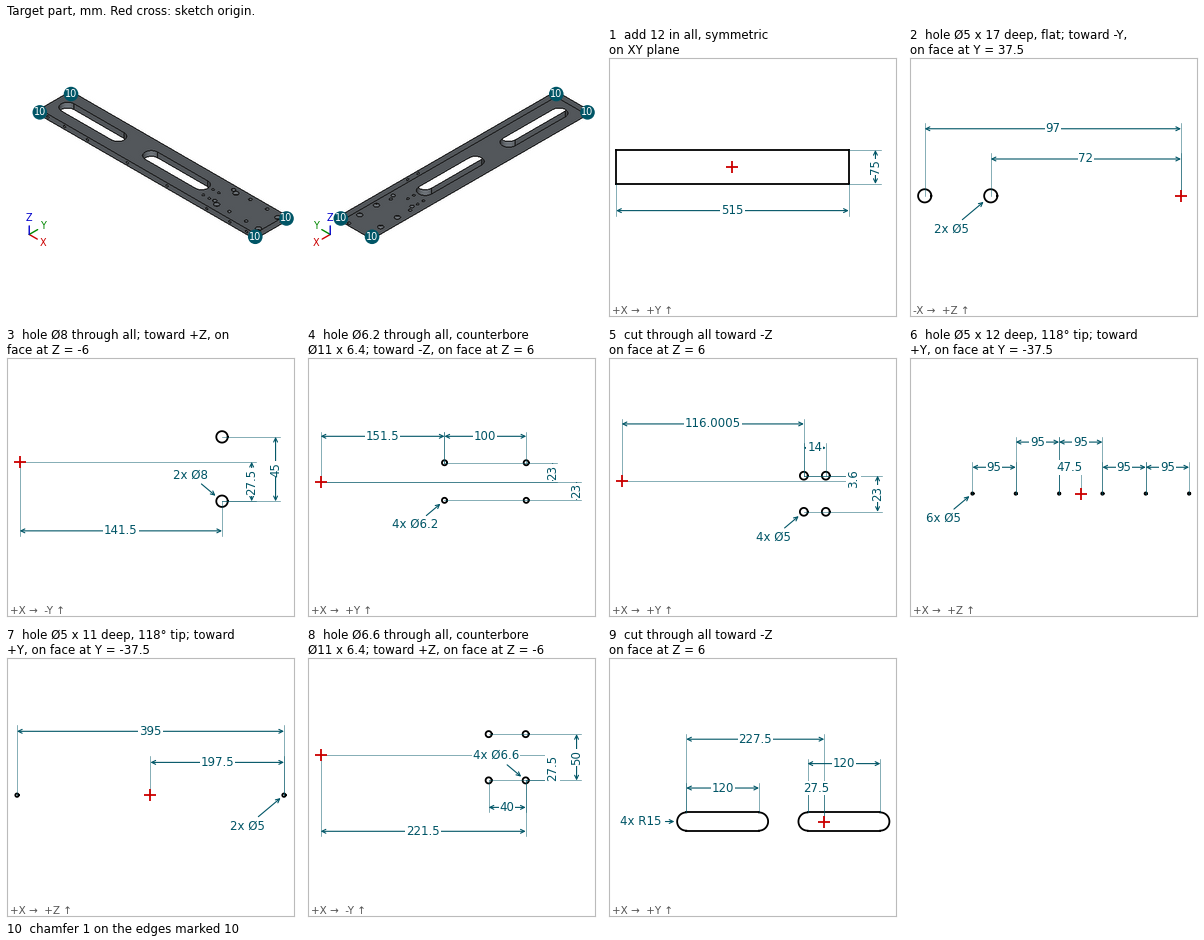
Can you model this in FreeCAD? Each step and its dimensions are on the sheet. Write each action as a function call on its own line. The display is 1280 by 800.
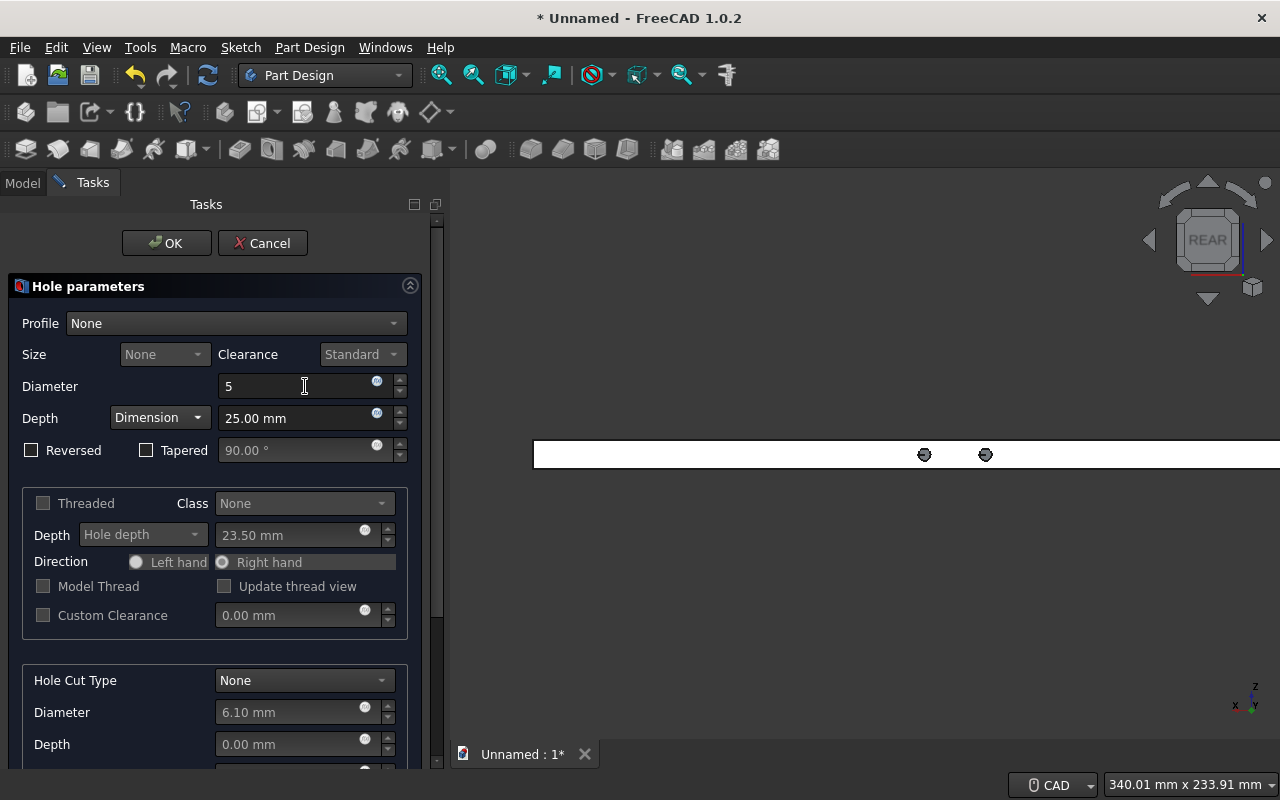
triple_click(305, 418)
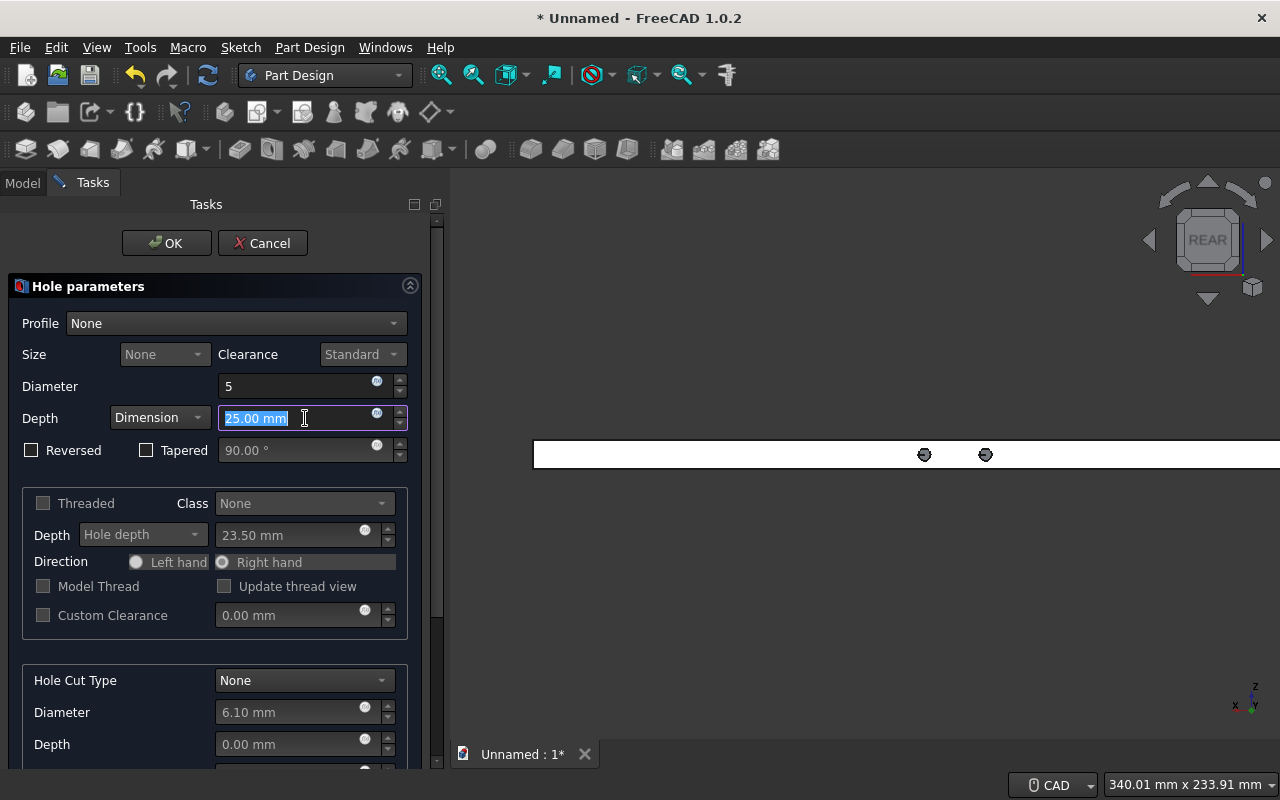
text(17)
key(Tab)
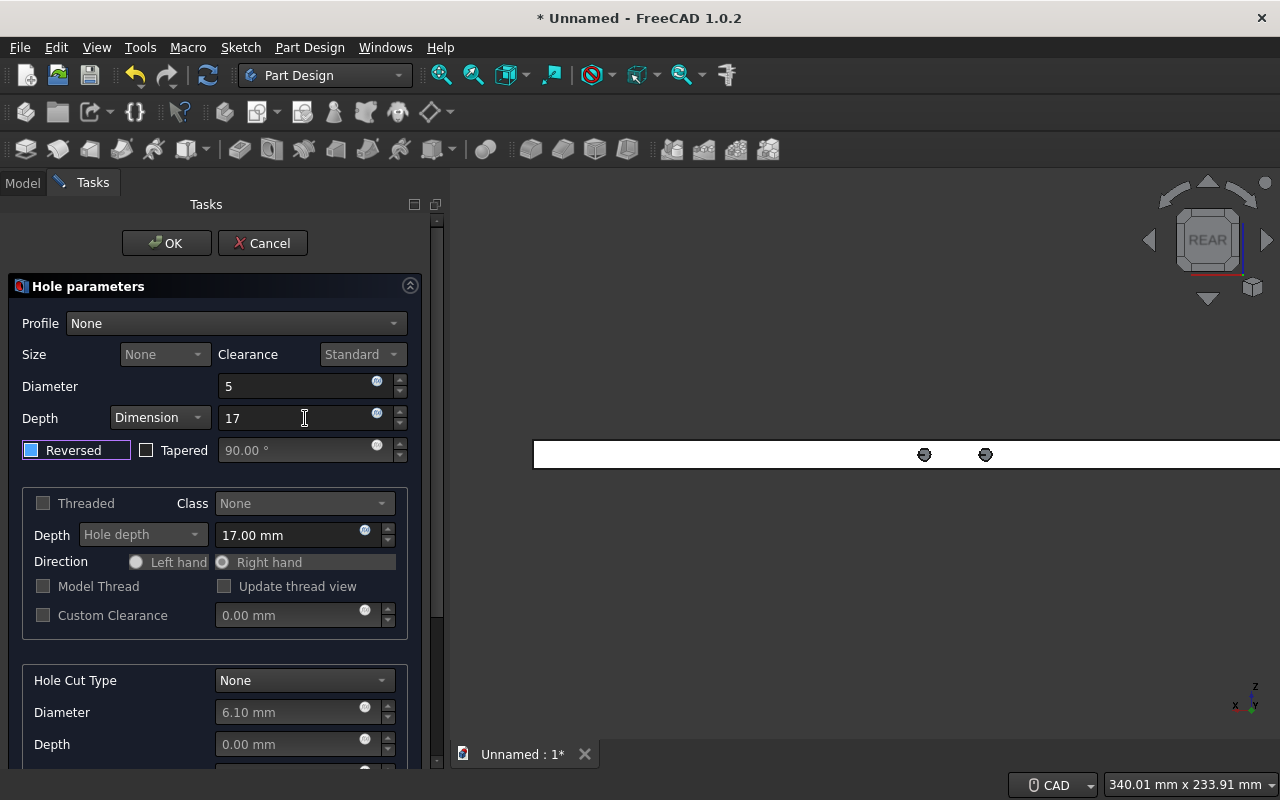
scroll(437, 491, down, 3)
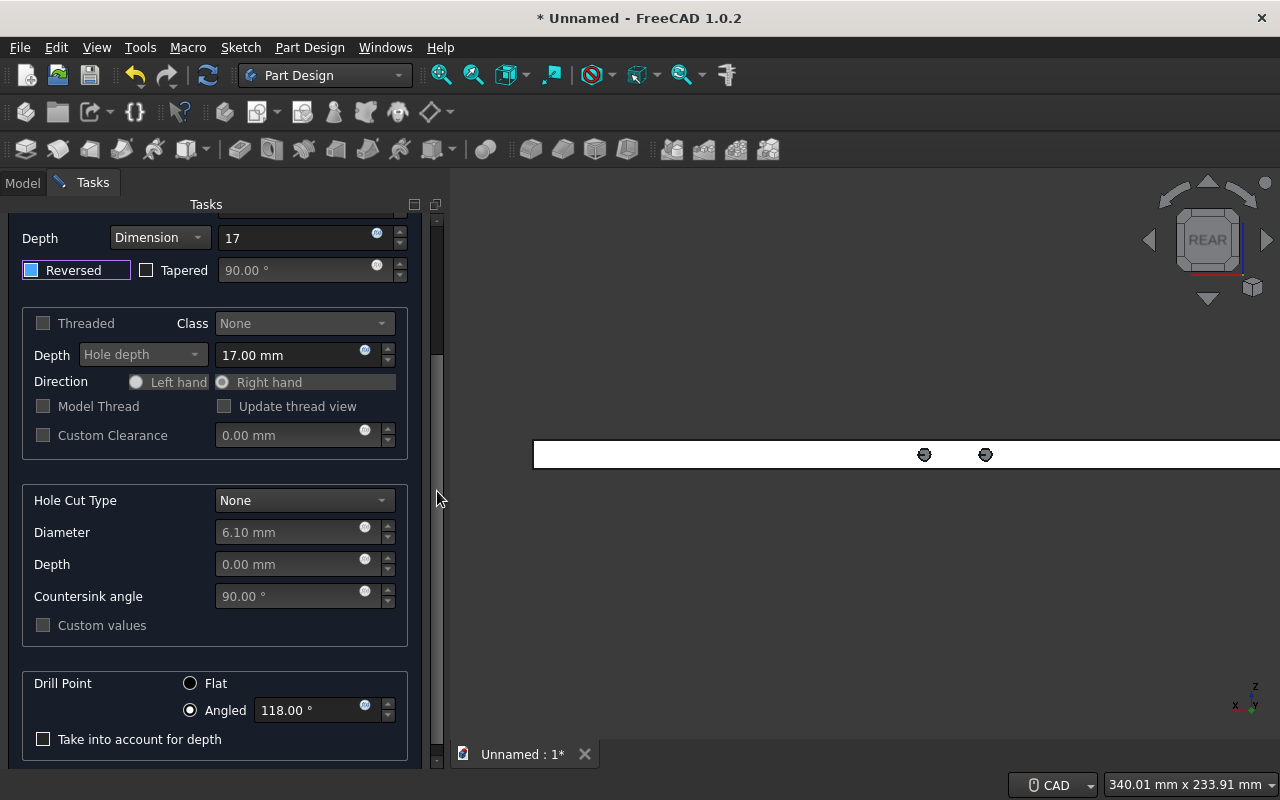
click(191, 683)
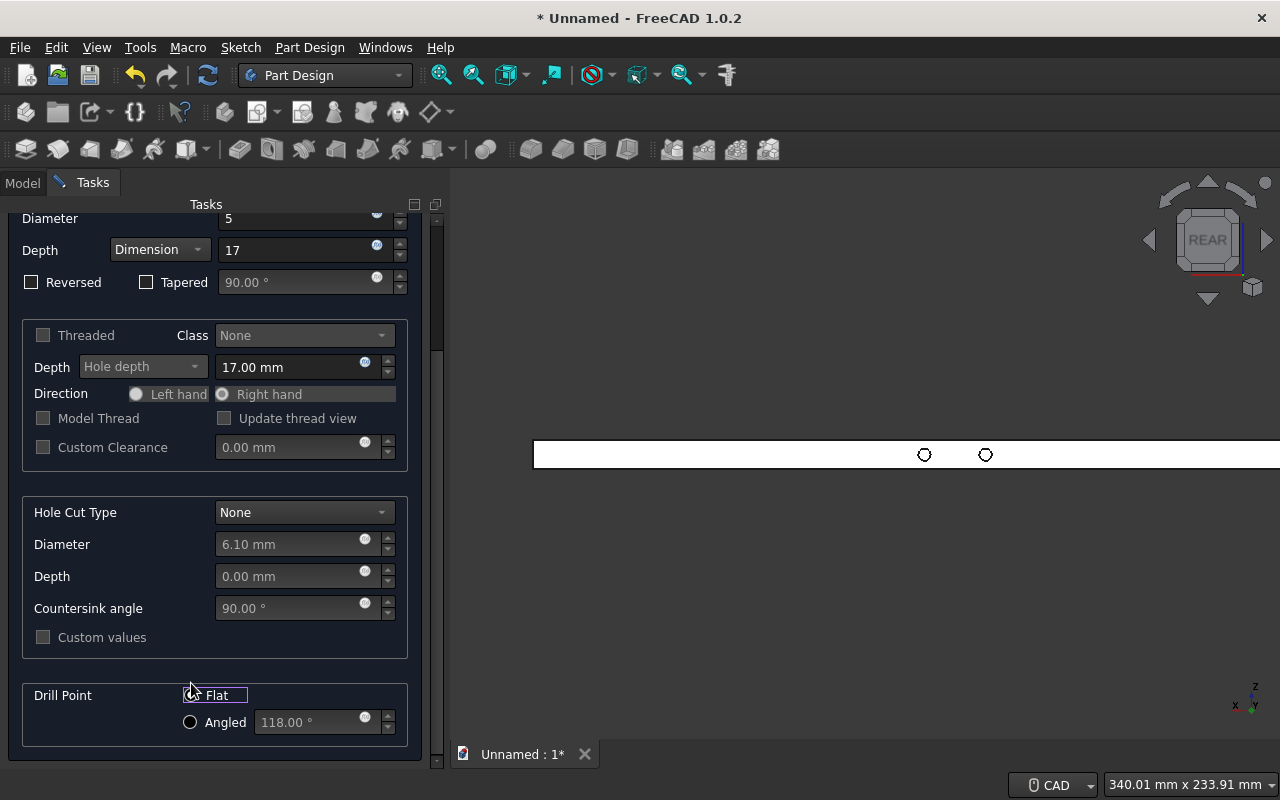
scroll(437, 491, up, 4)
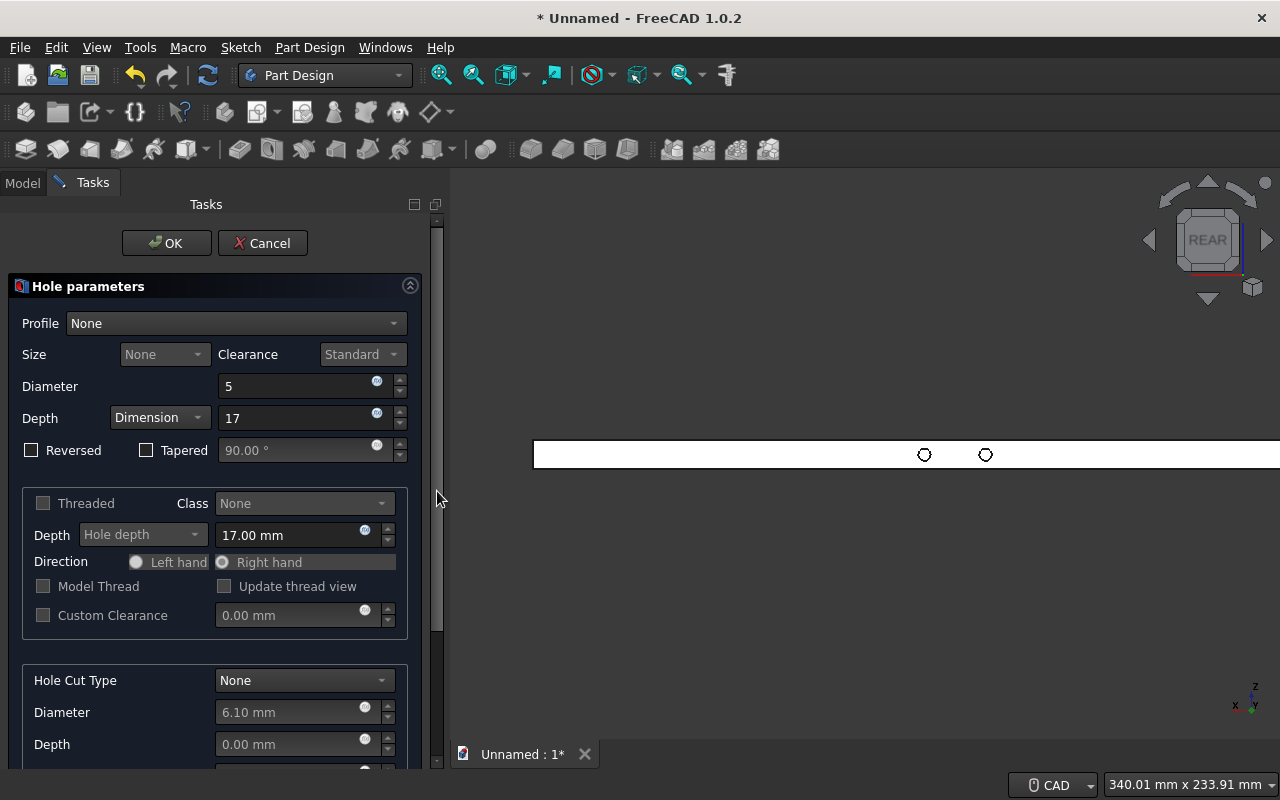
click(167, 243)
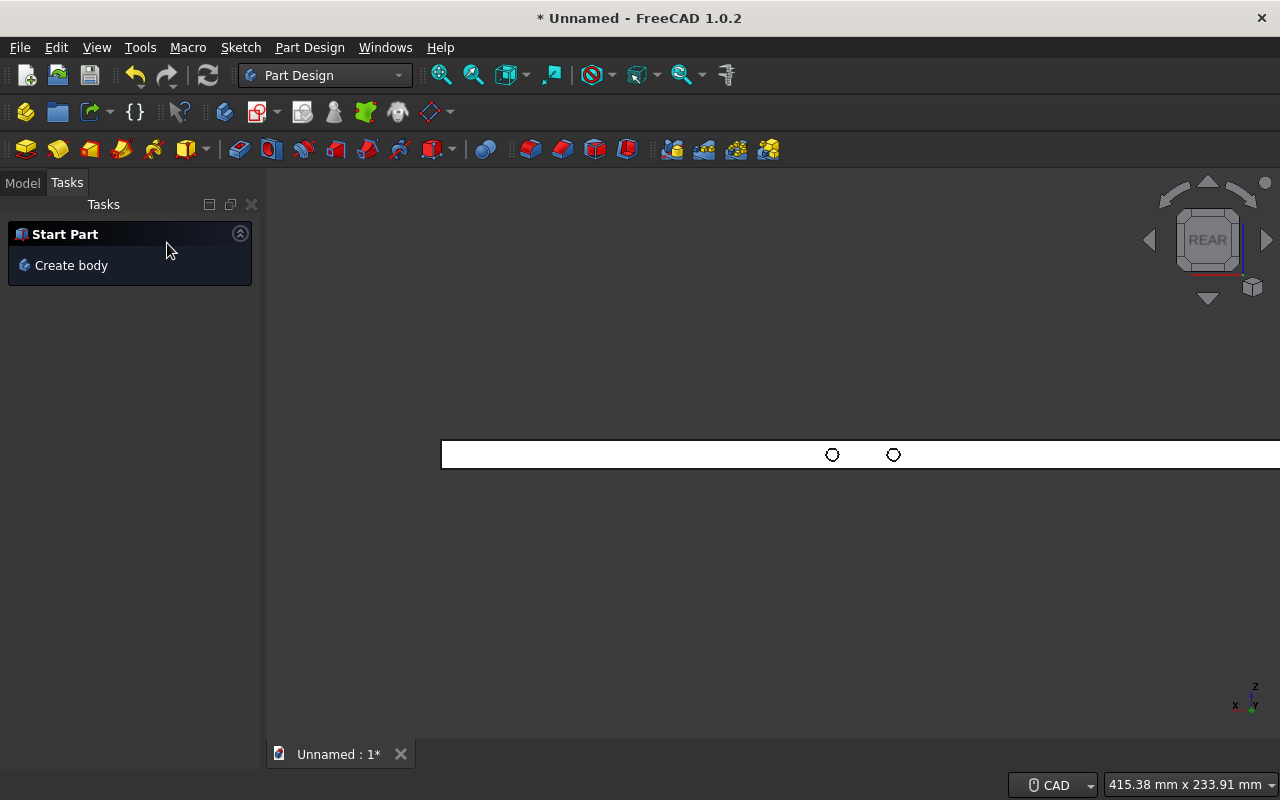
key(v)
key(f)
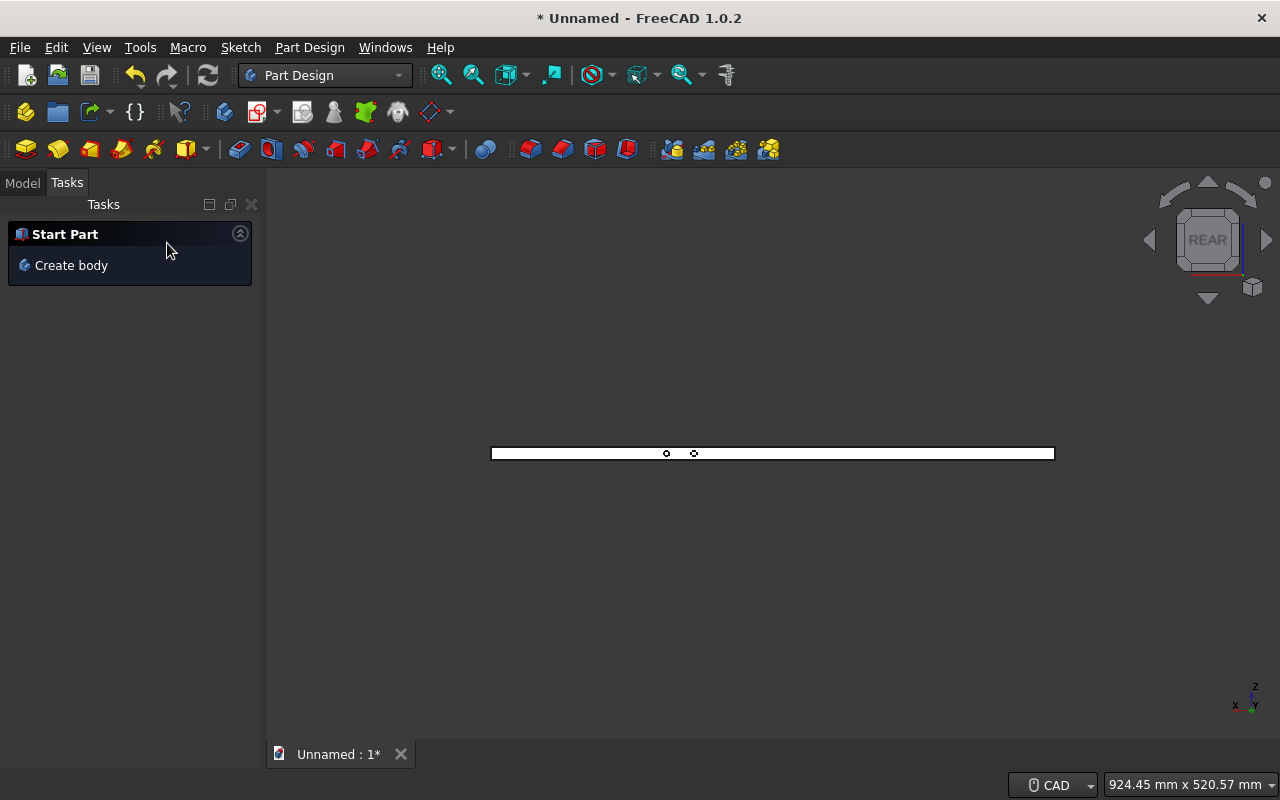
key(5)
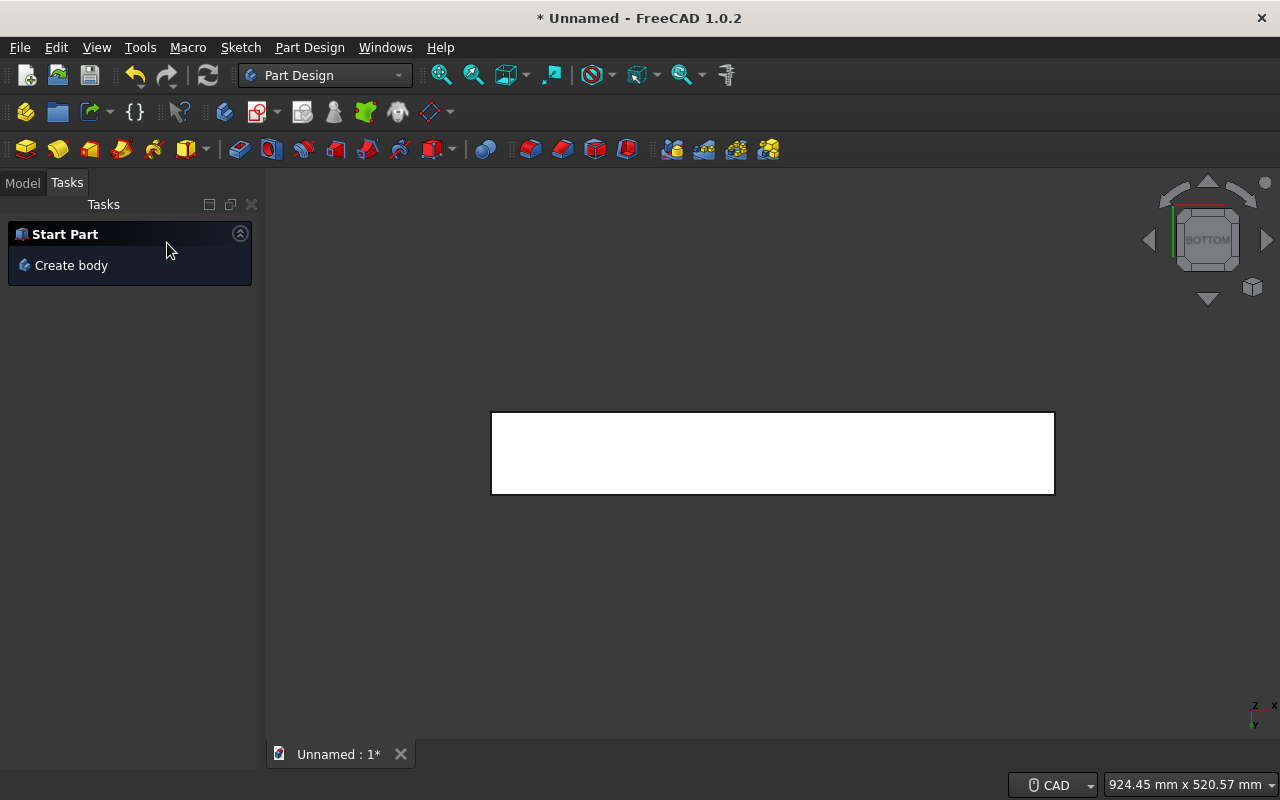
click(934, 452)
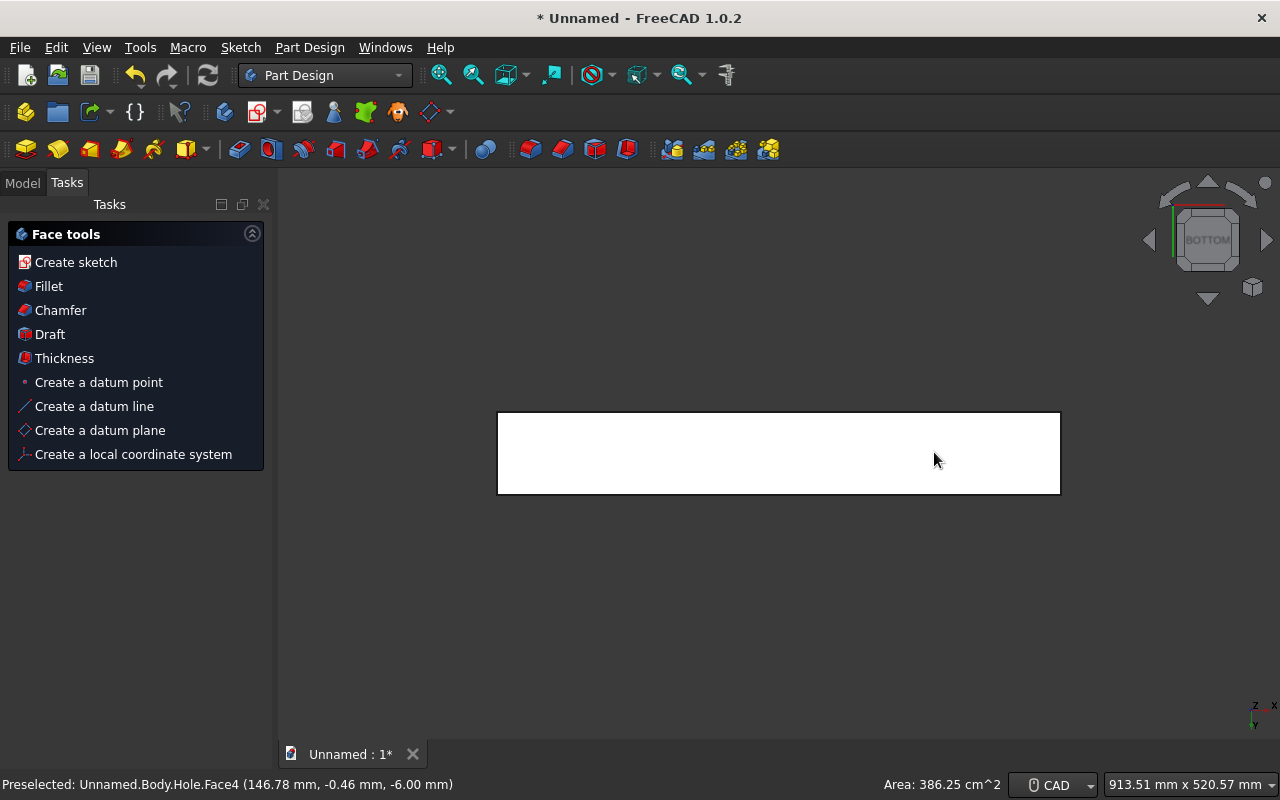
click(258, 112)